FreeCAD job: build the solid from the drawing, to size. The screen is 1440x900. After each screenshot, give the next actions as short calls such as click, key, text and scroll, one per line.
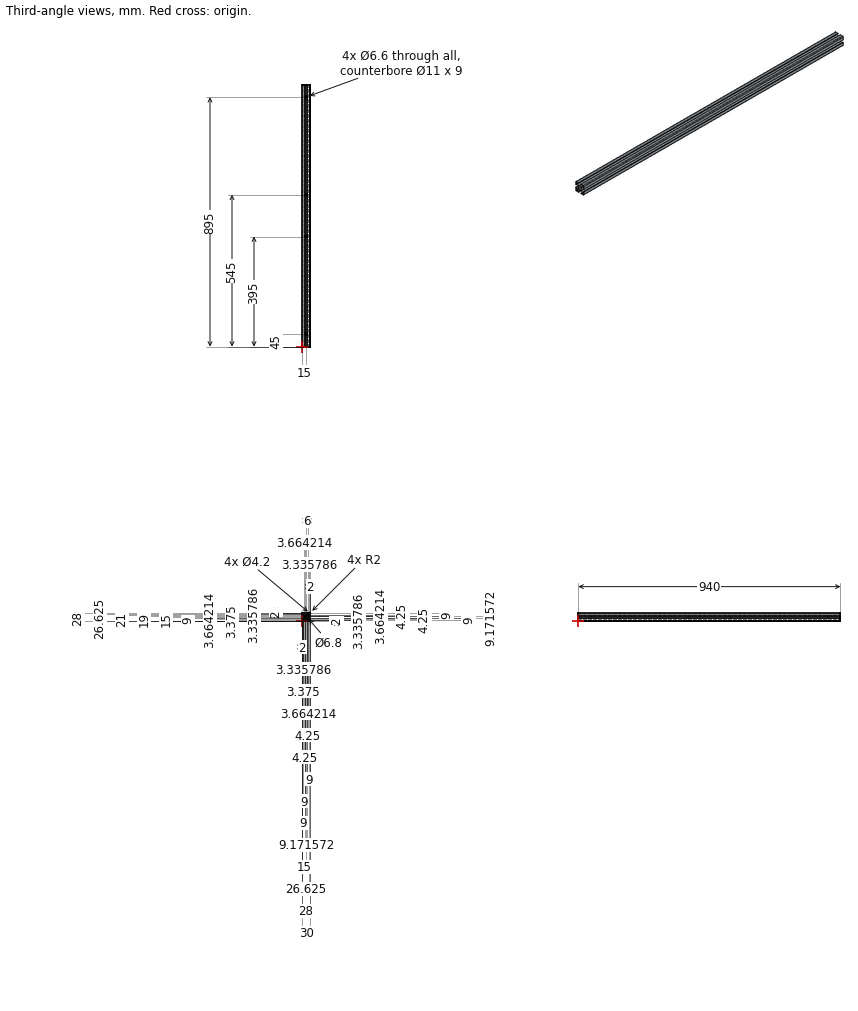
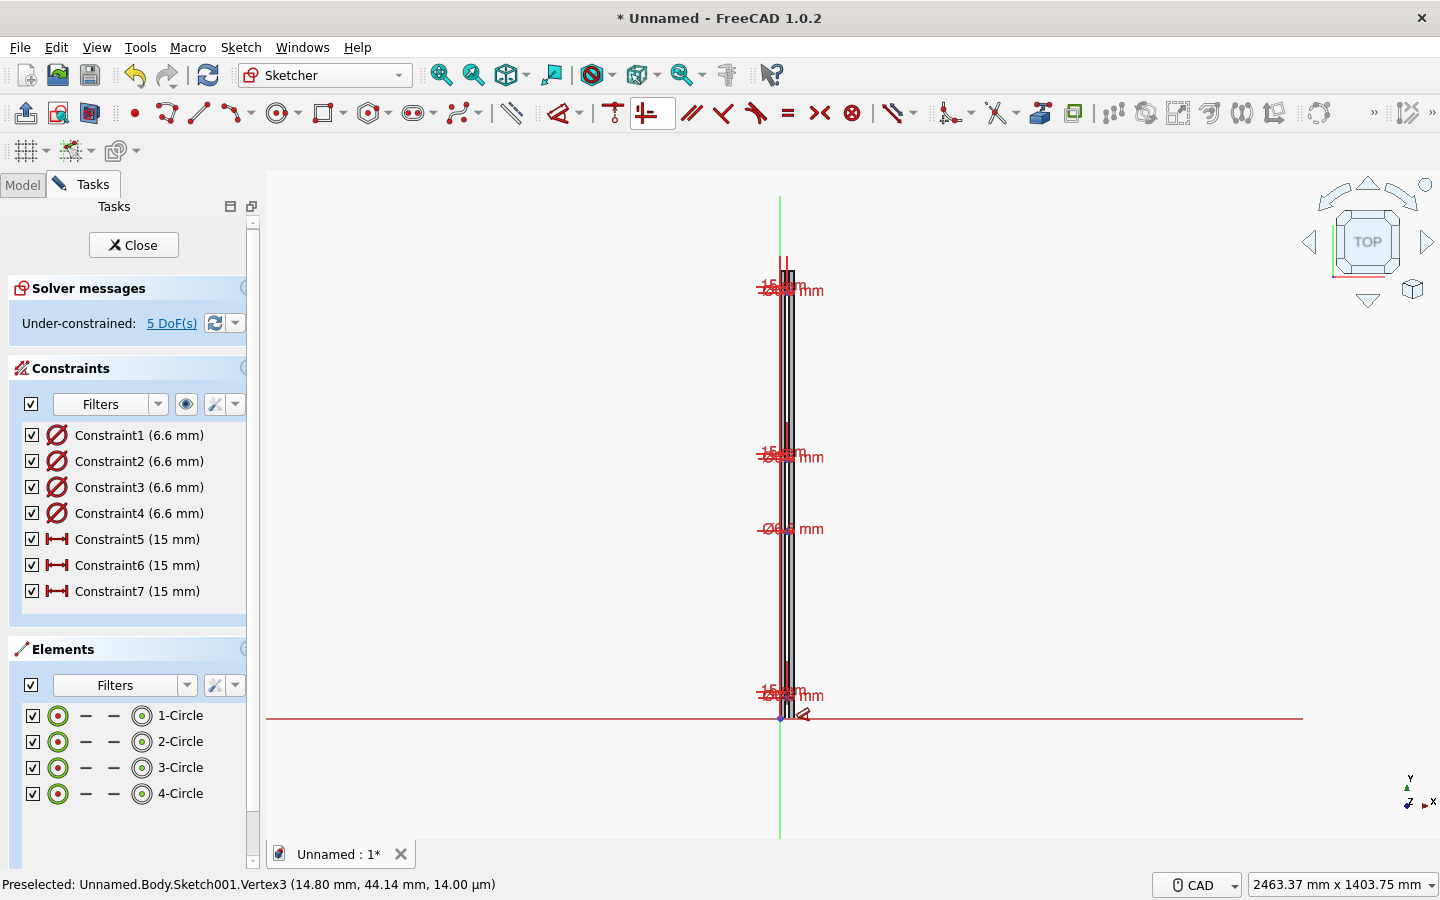
scroll(787, 698, up, 4)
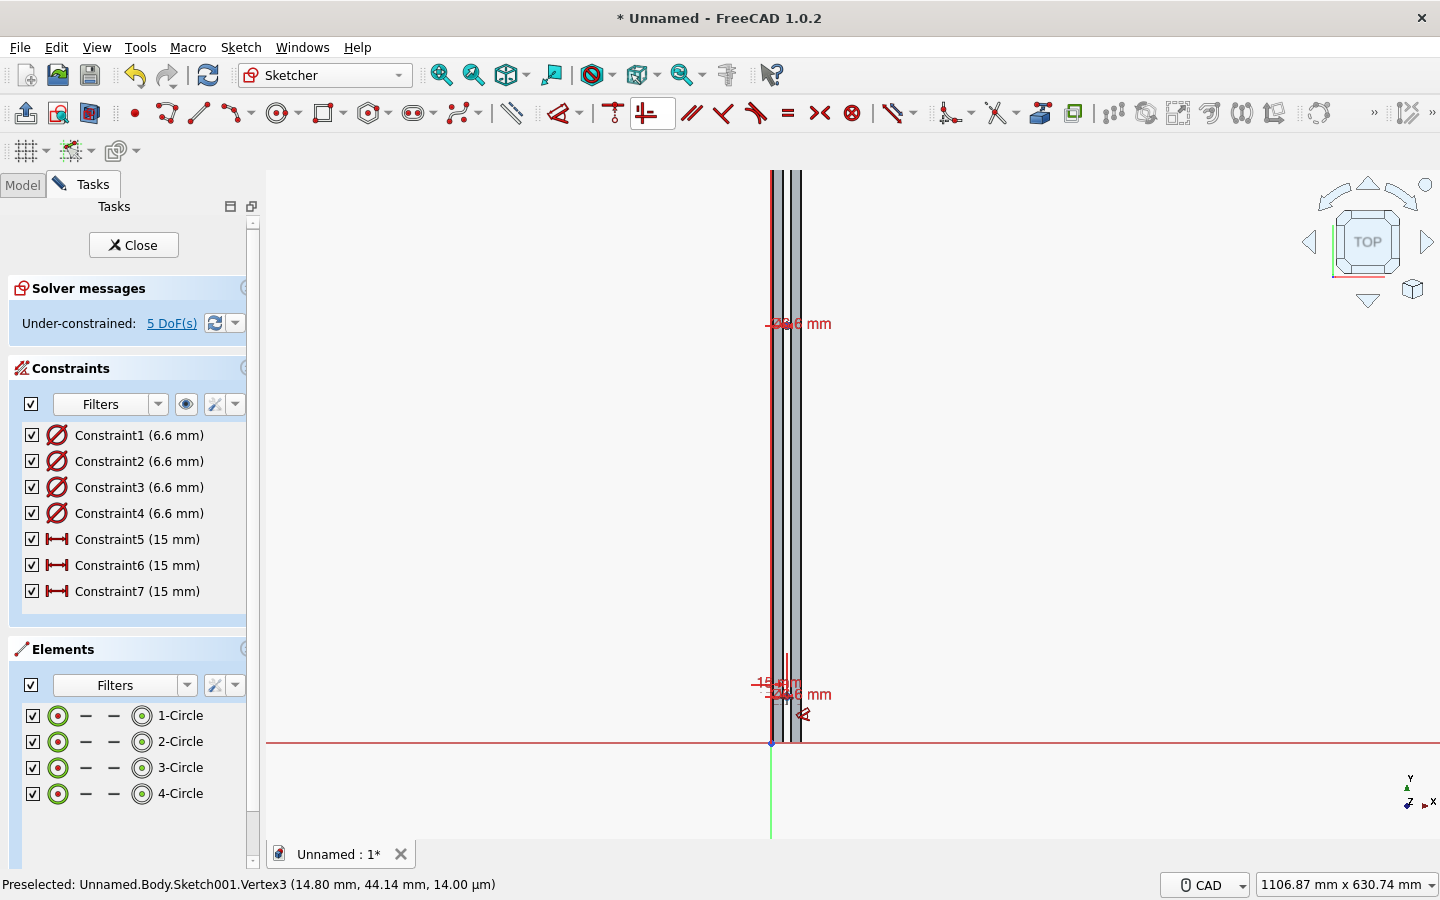
click(787, 697)
click(737, 720)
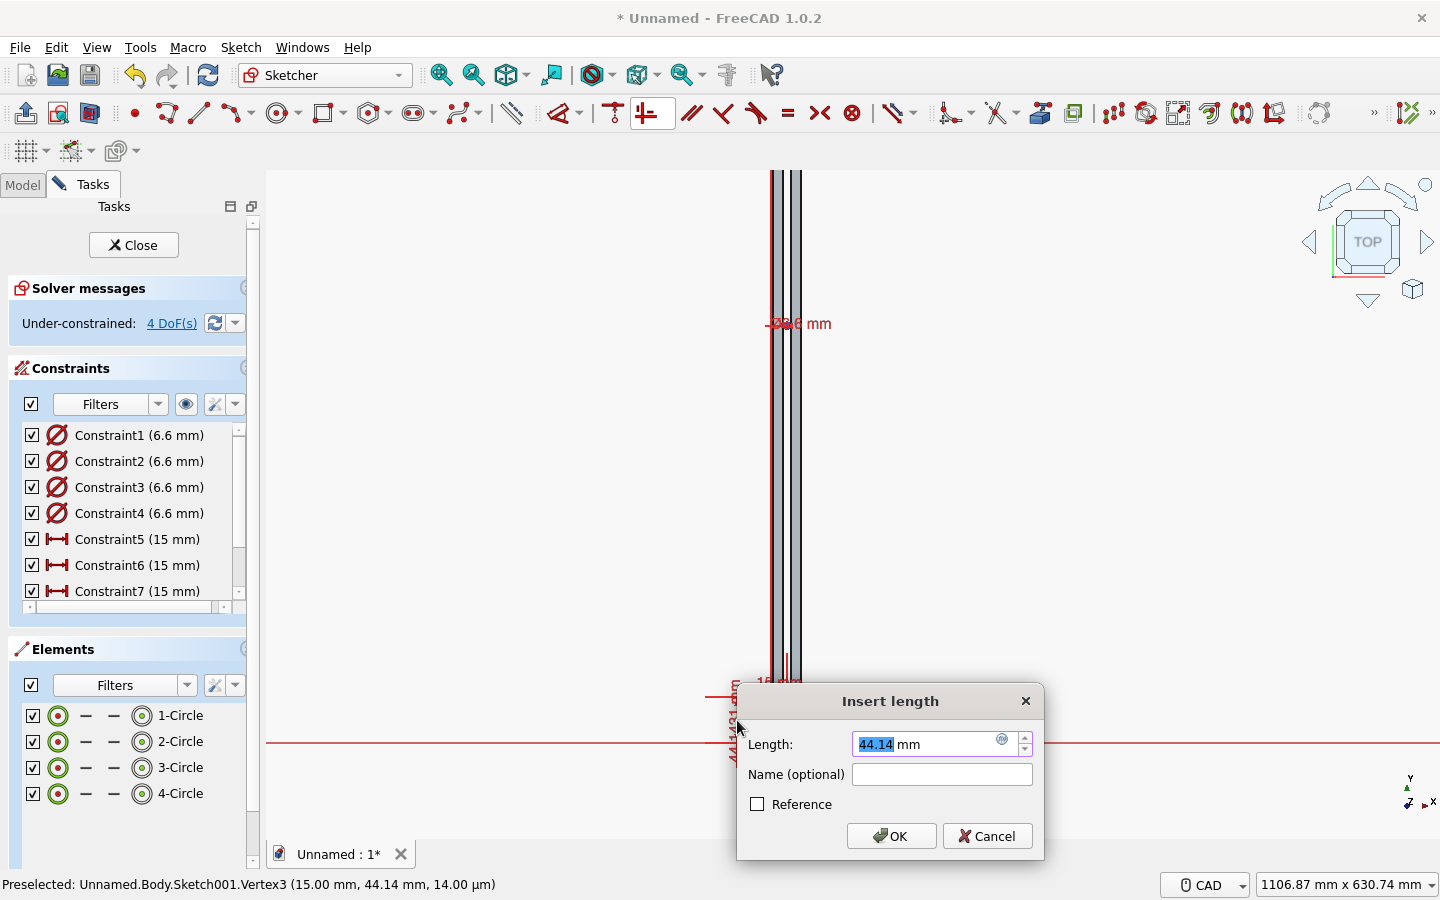
text(45)
key(Return)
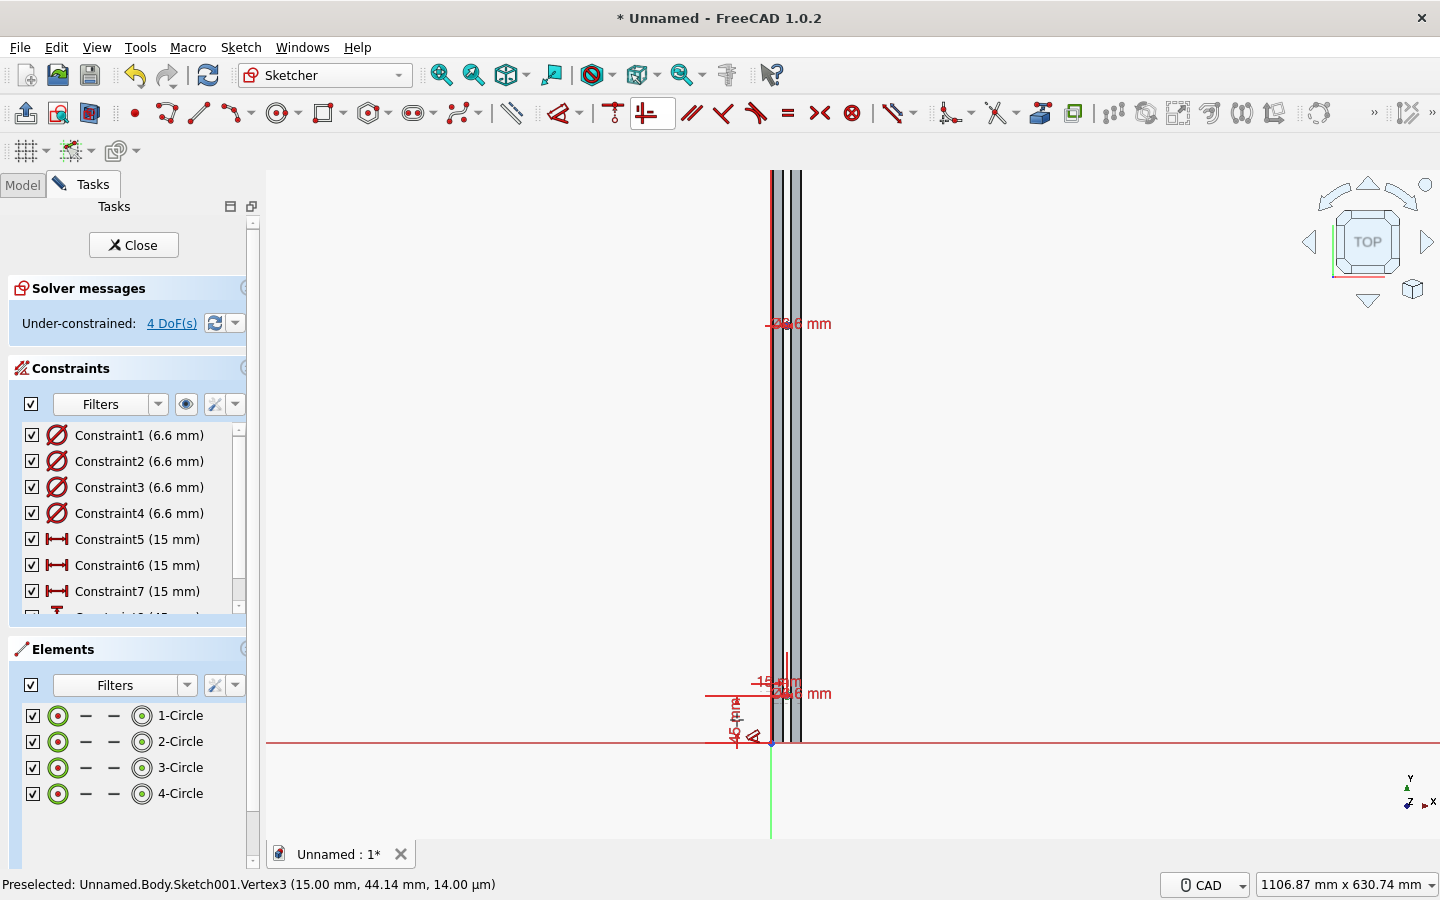
scroll(787, 326, up, 5)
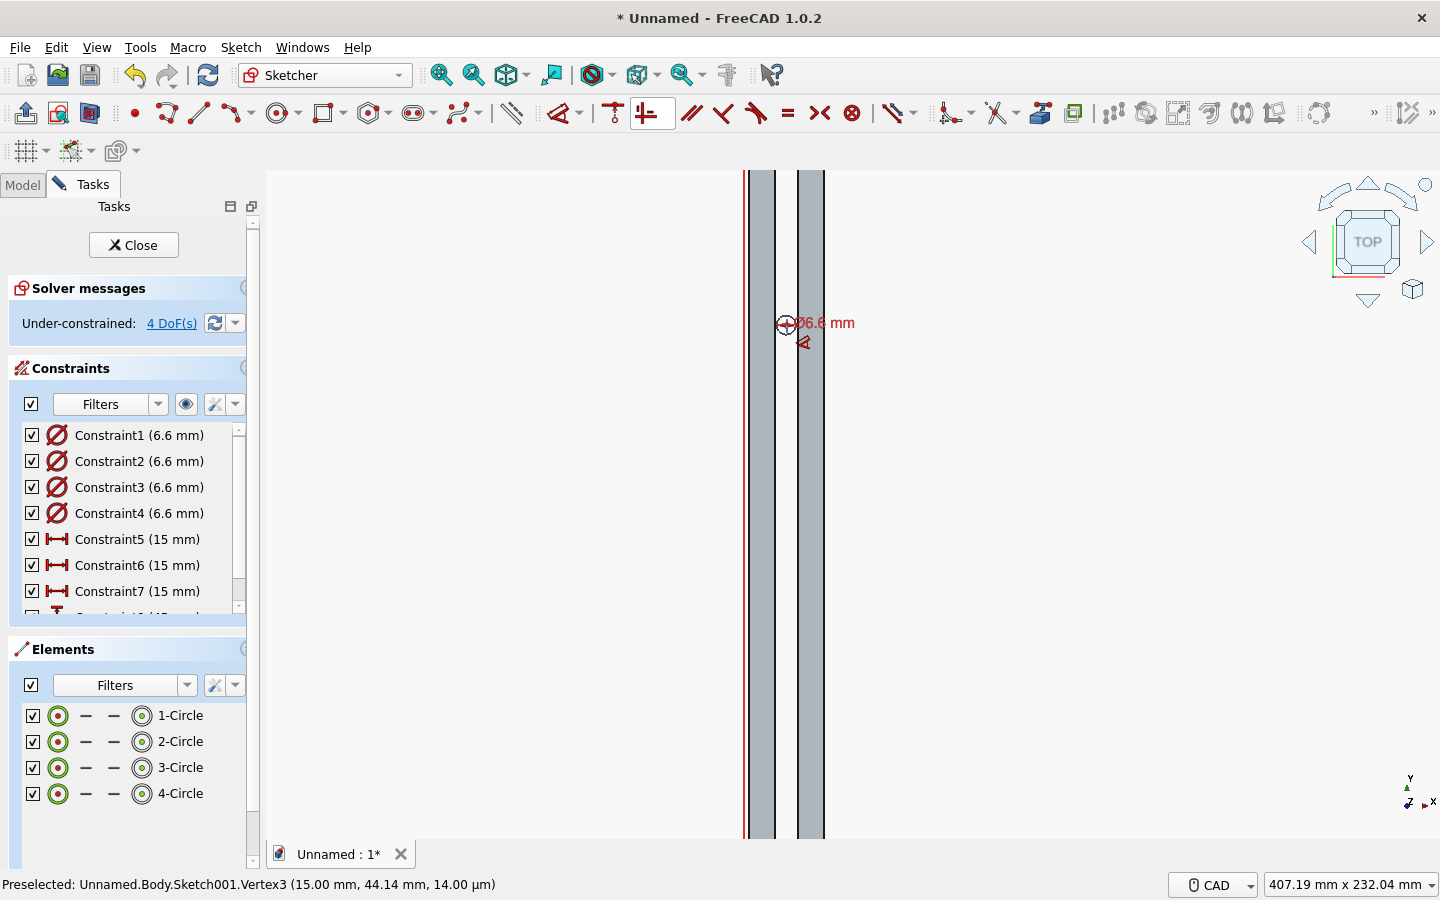
click(786, 325)
click(765, 291)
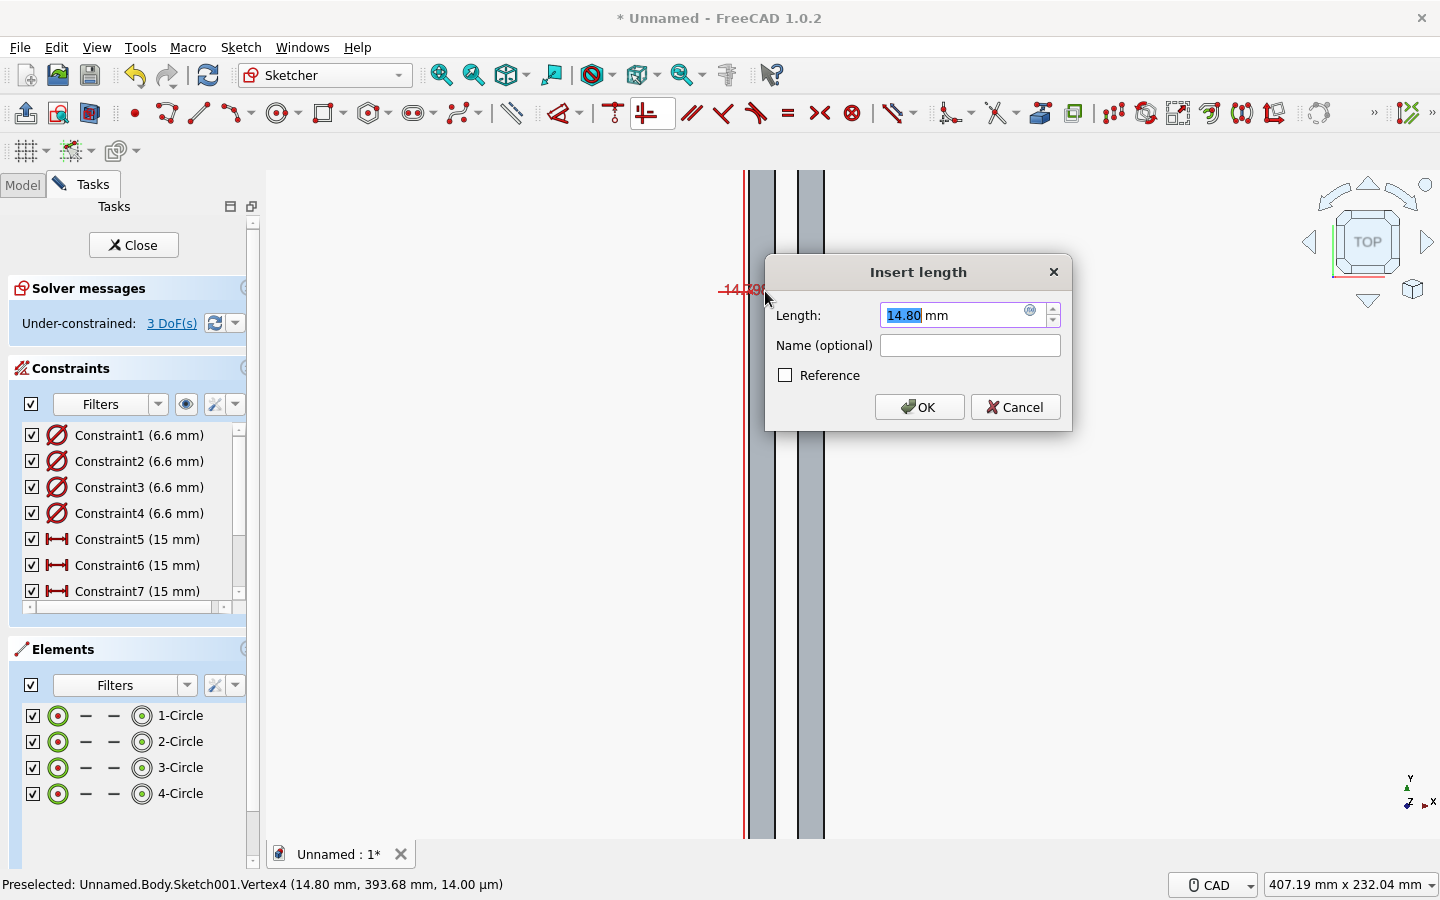
text(15)
key(Return)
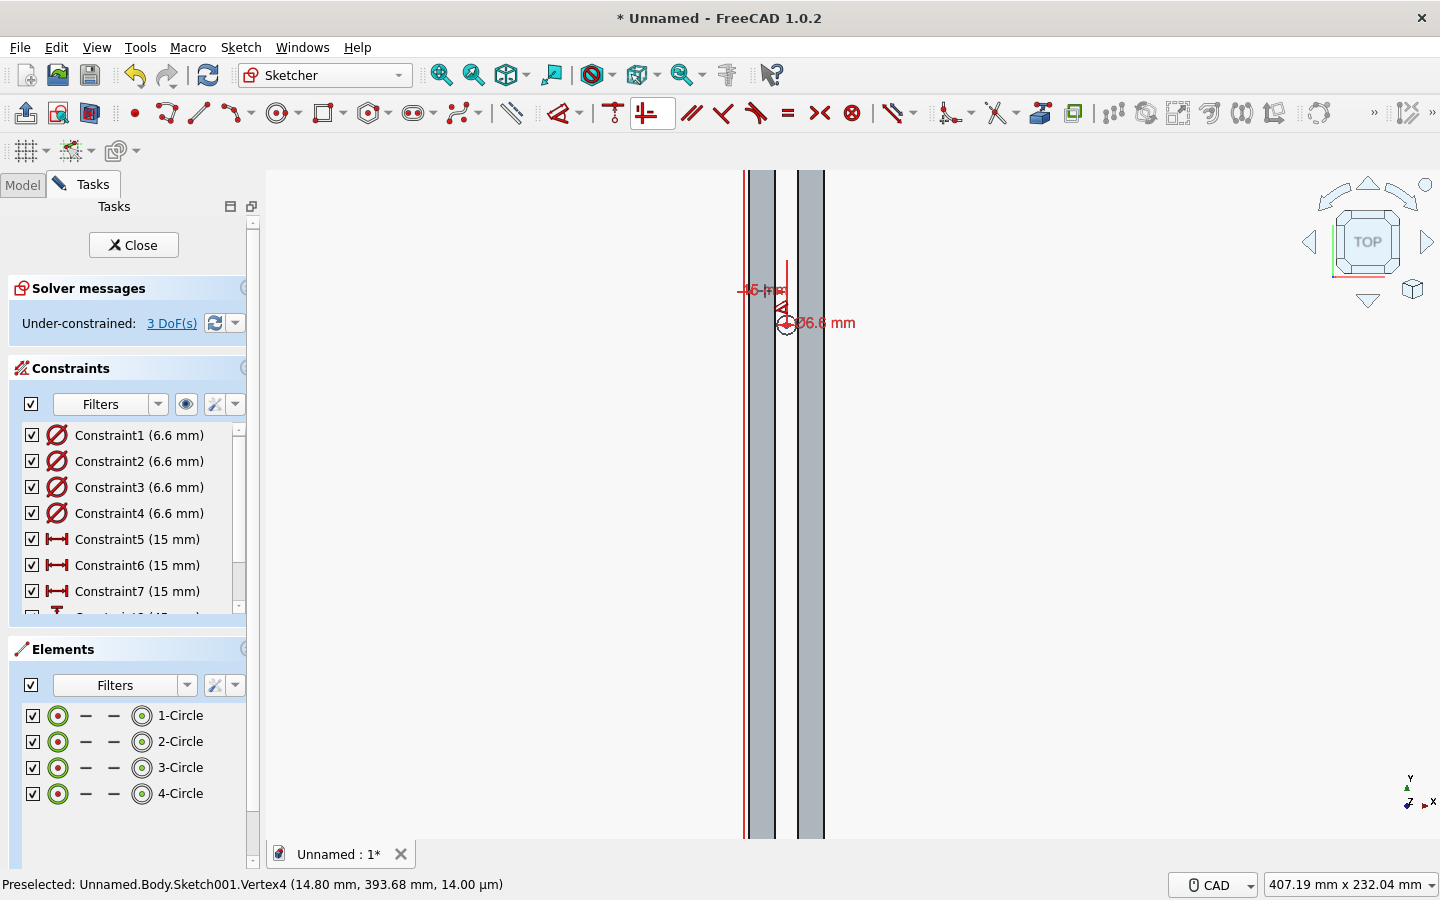
scroll(787, 572, down, 9)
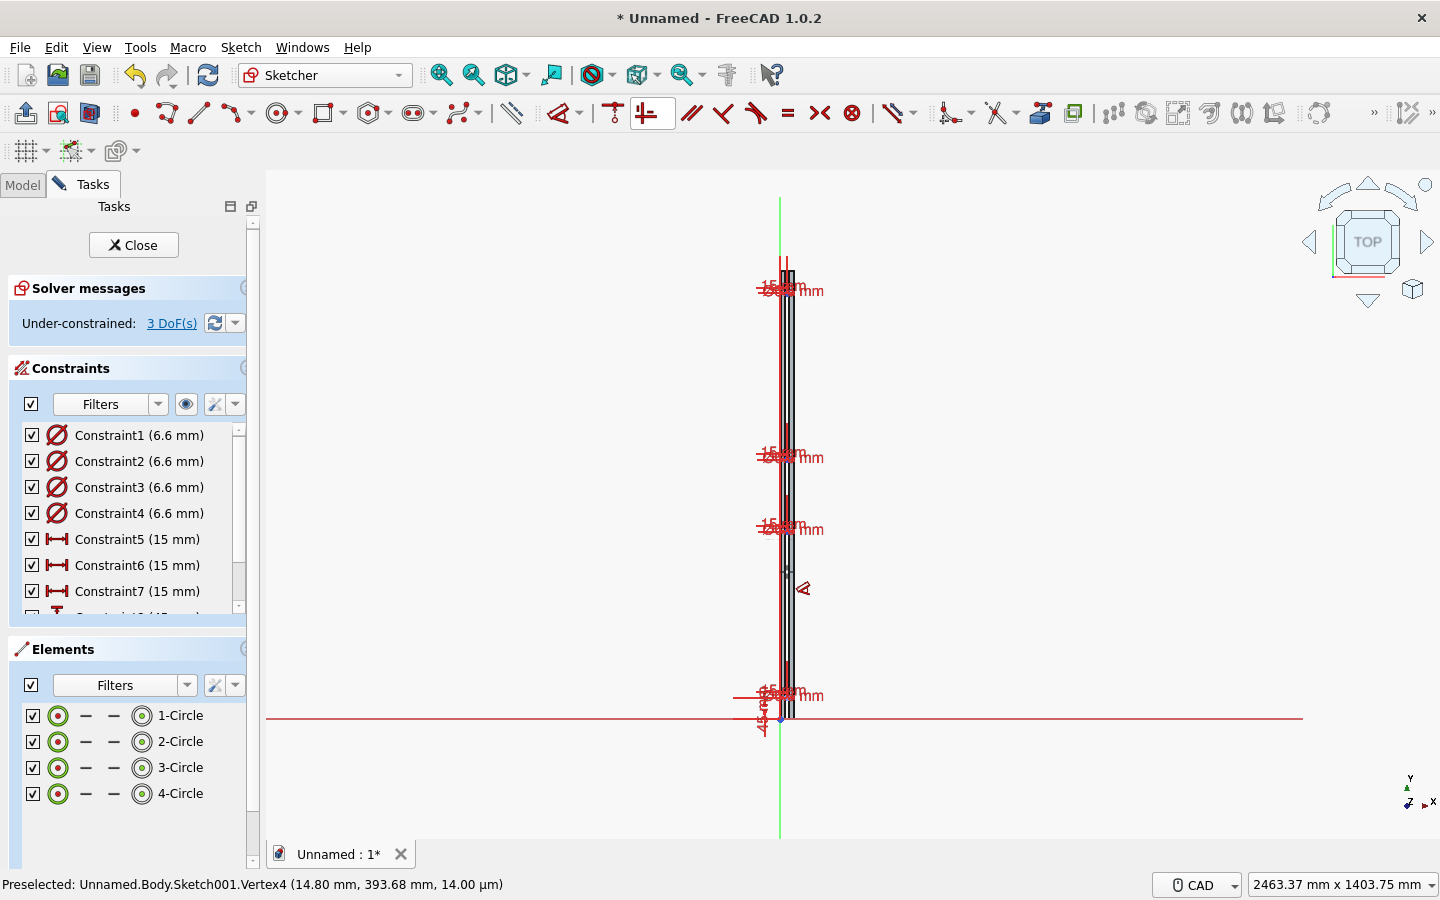
click(787, 293)
click(746, 408)